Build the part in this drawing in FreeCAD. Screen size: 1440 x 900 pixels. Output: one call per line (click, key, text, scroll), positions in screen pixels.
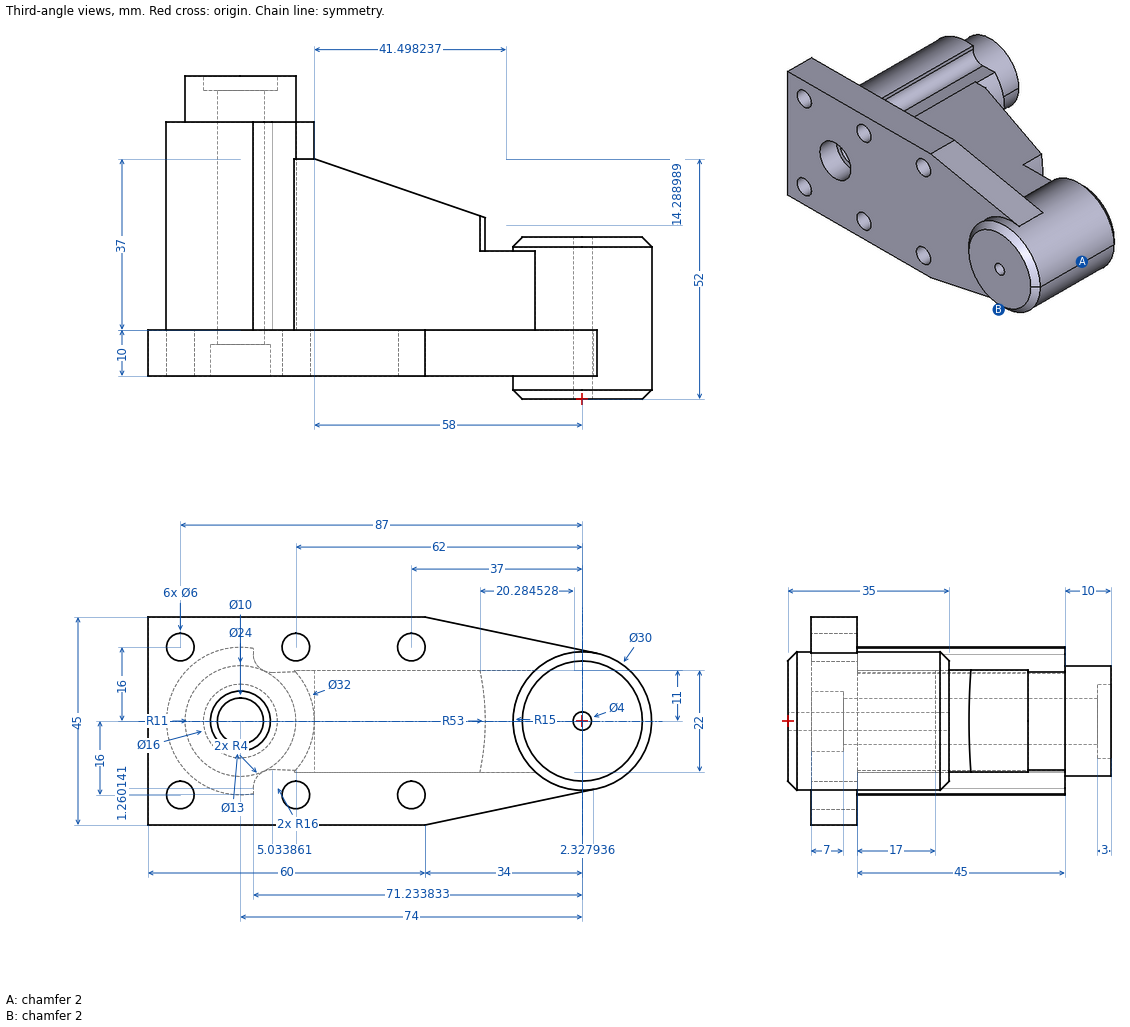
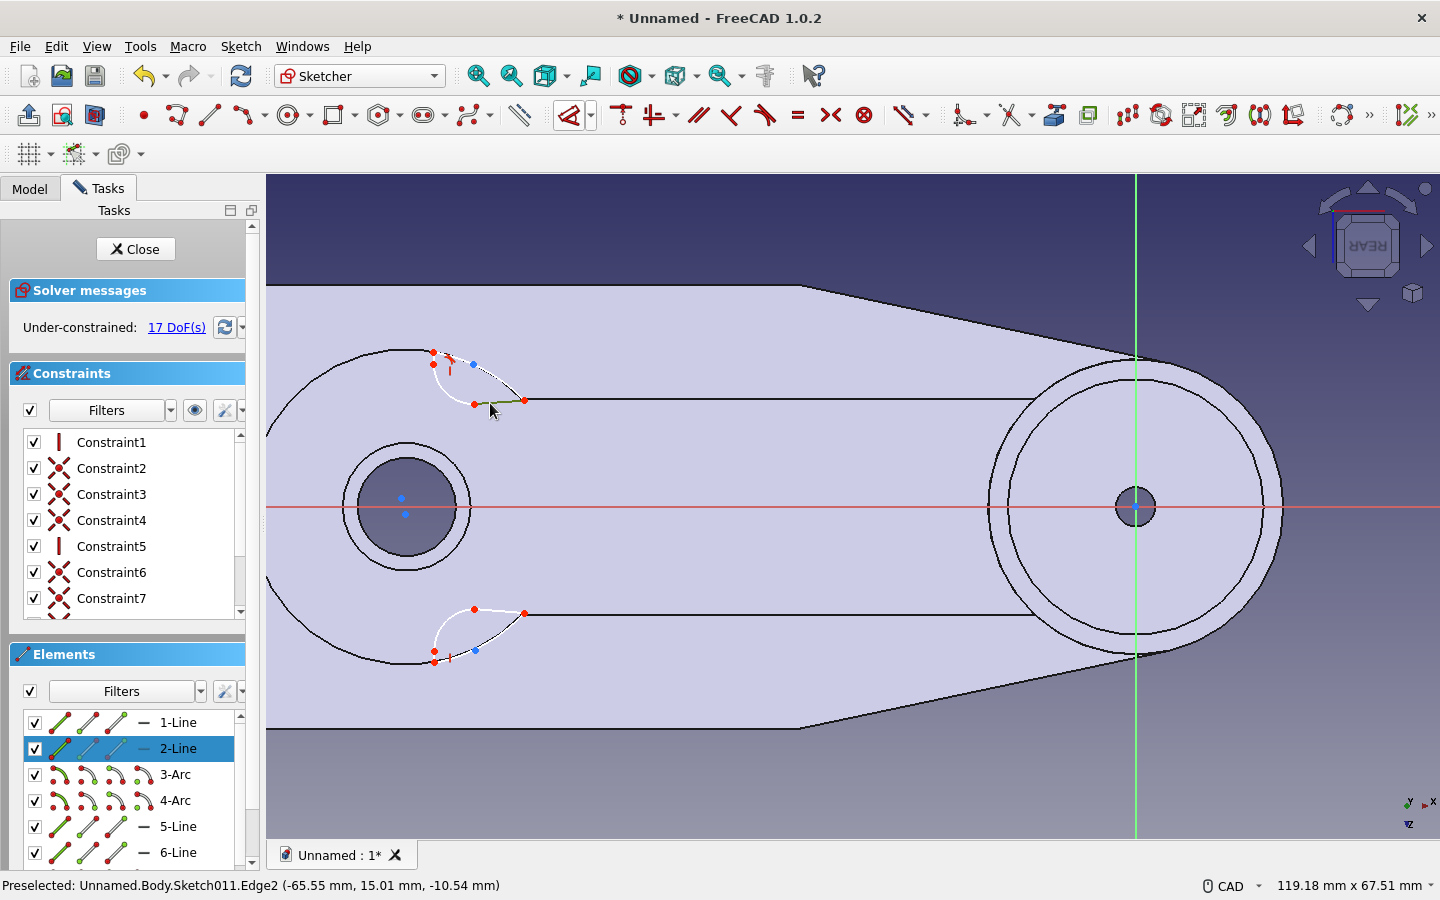
click(438, 383)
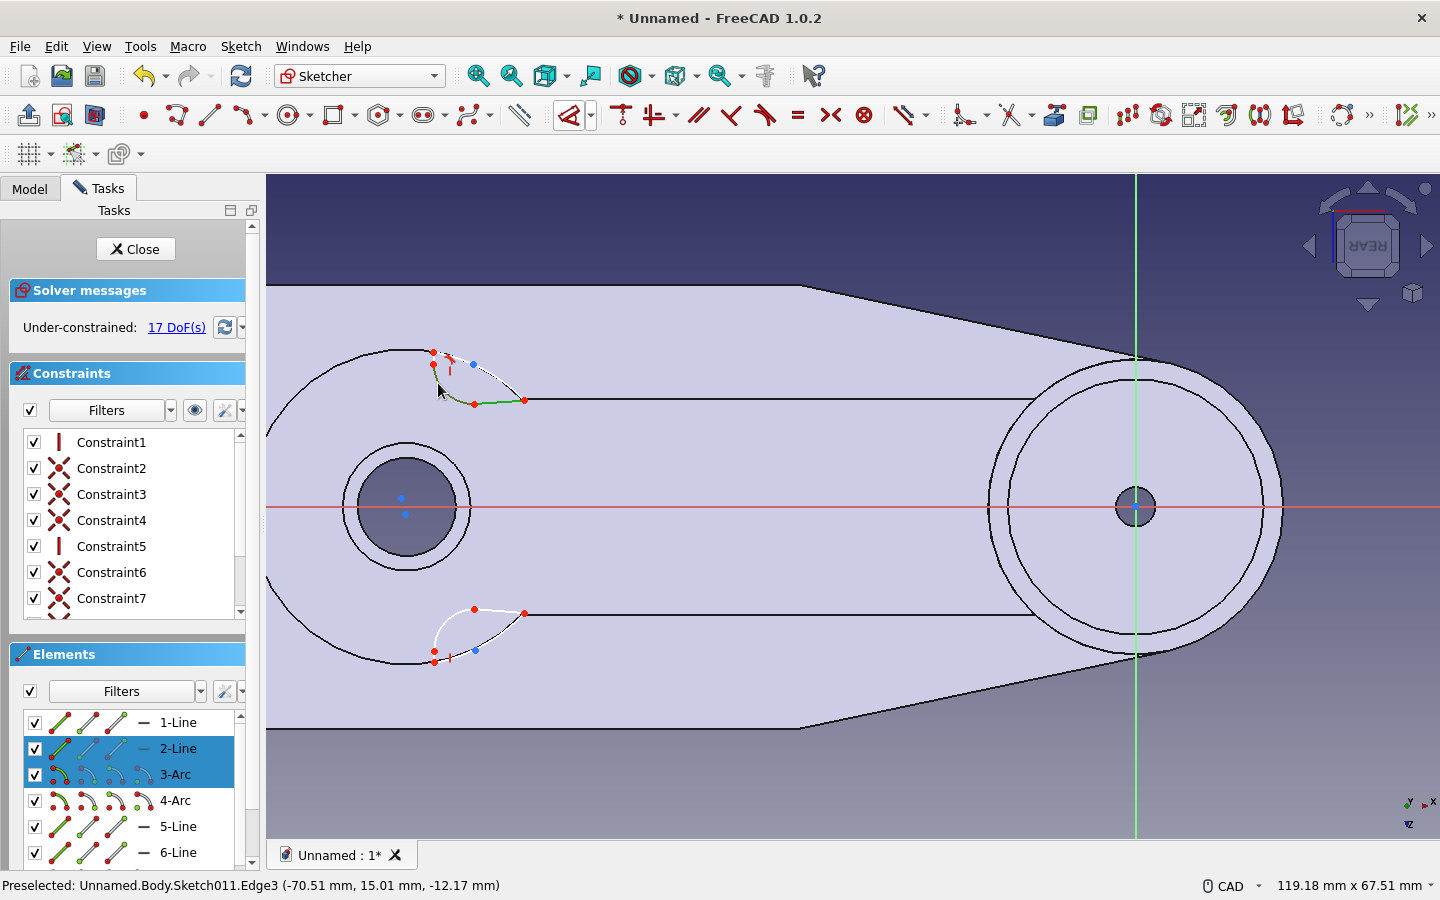
click(765, 116)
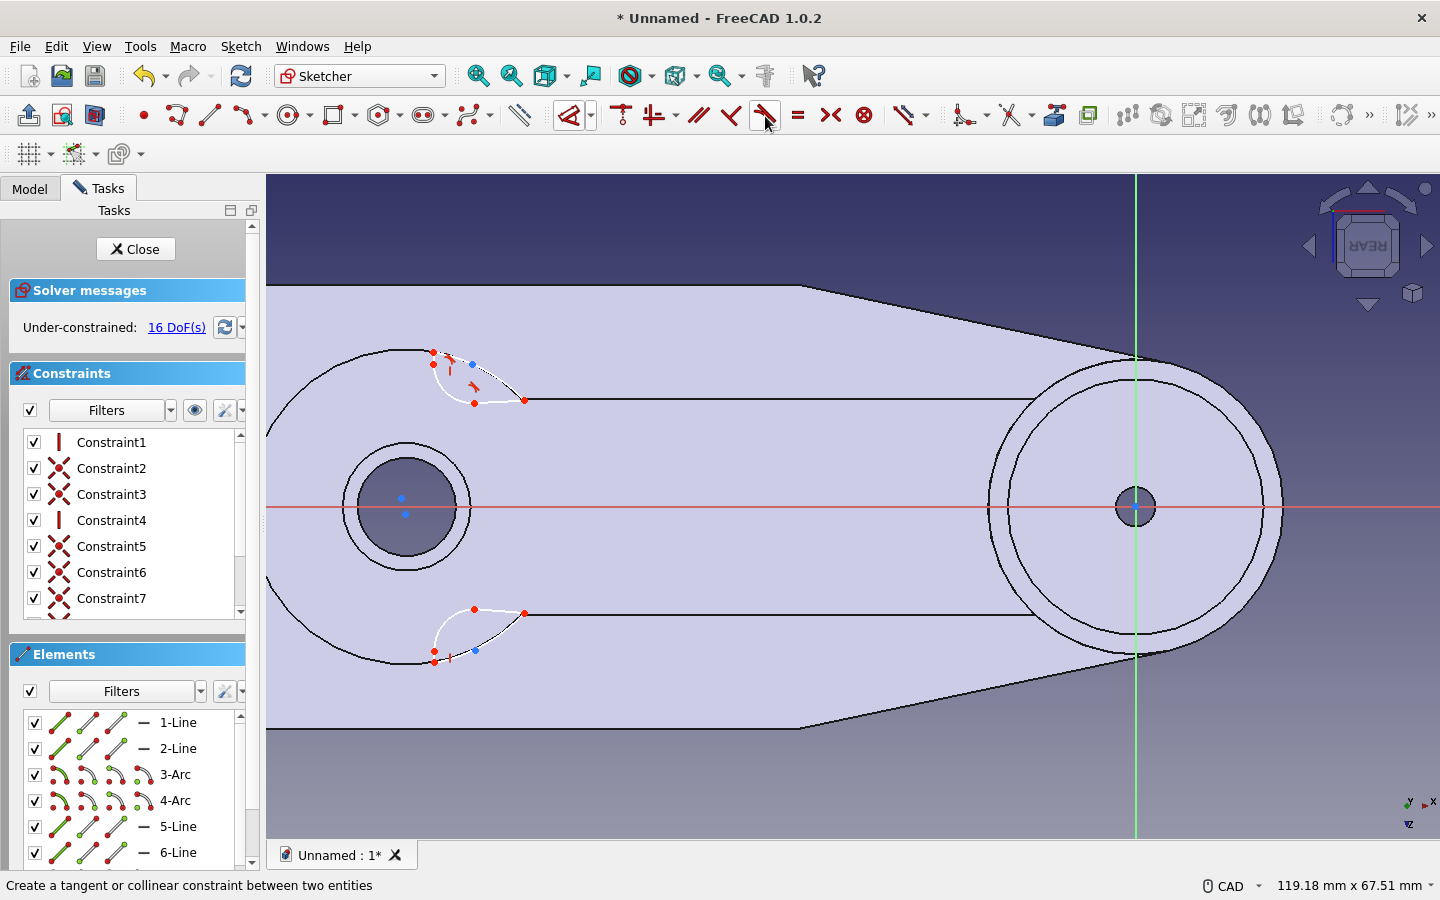
click(509, 612)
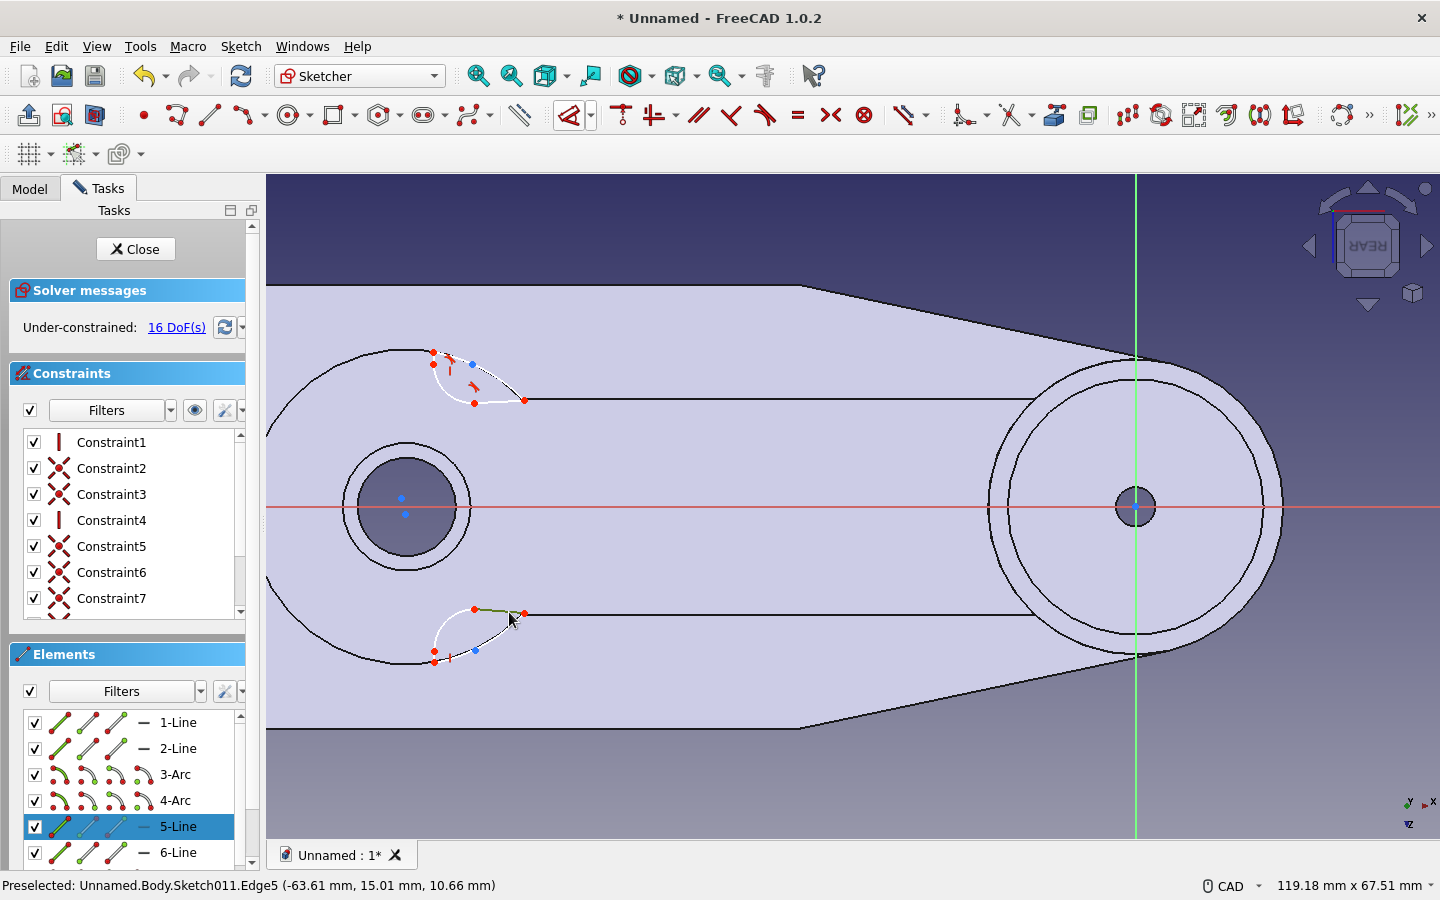
click(456, 614)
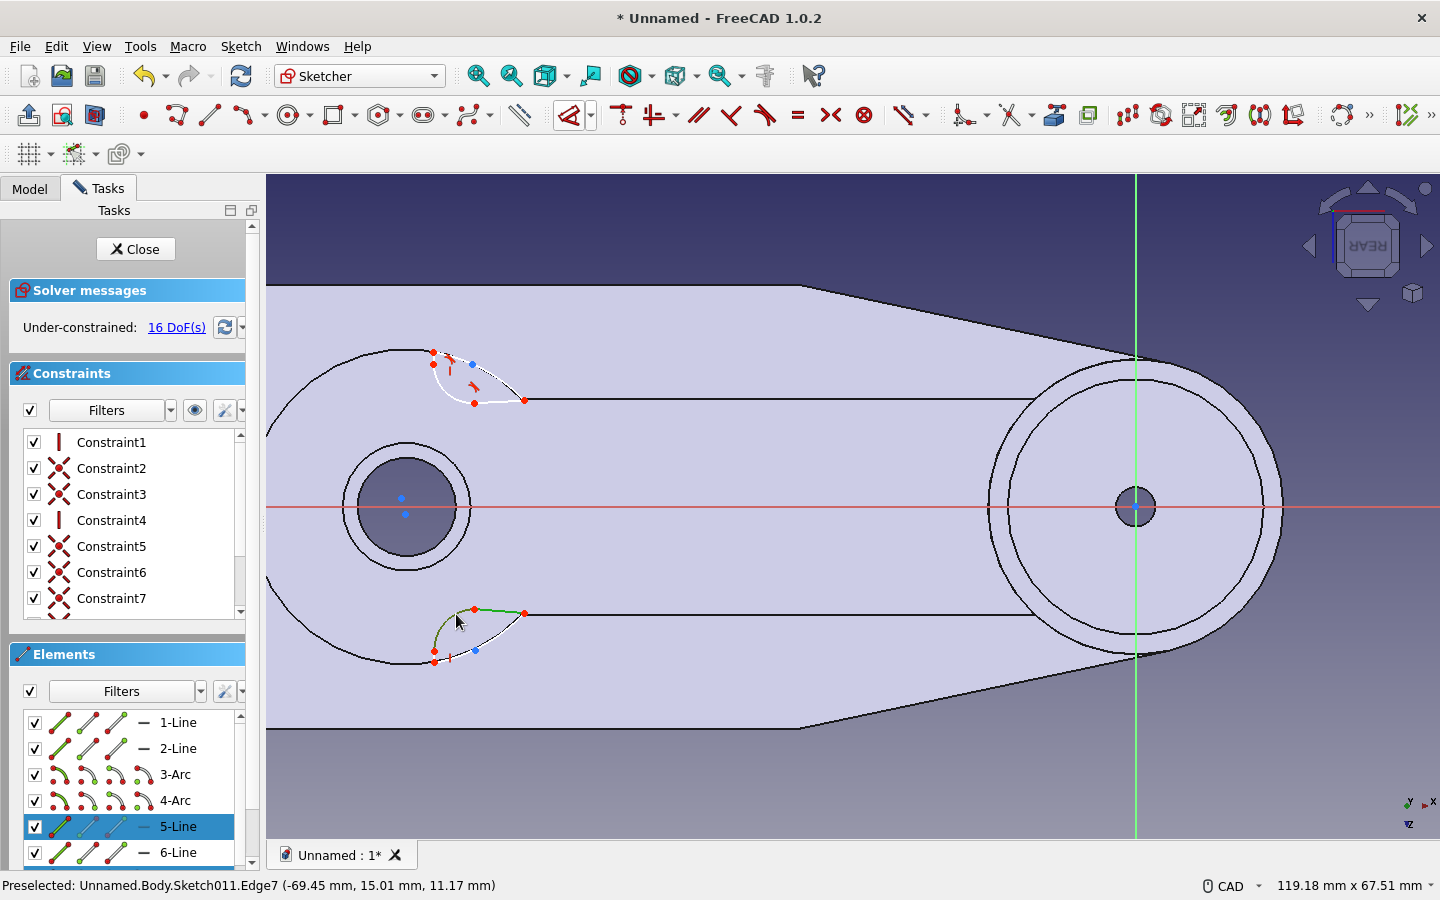
click(765, 116)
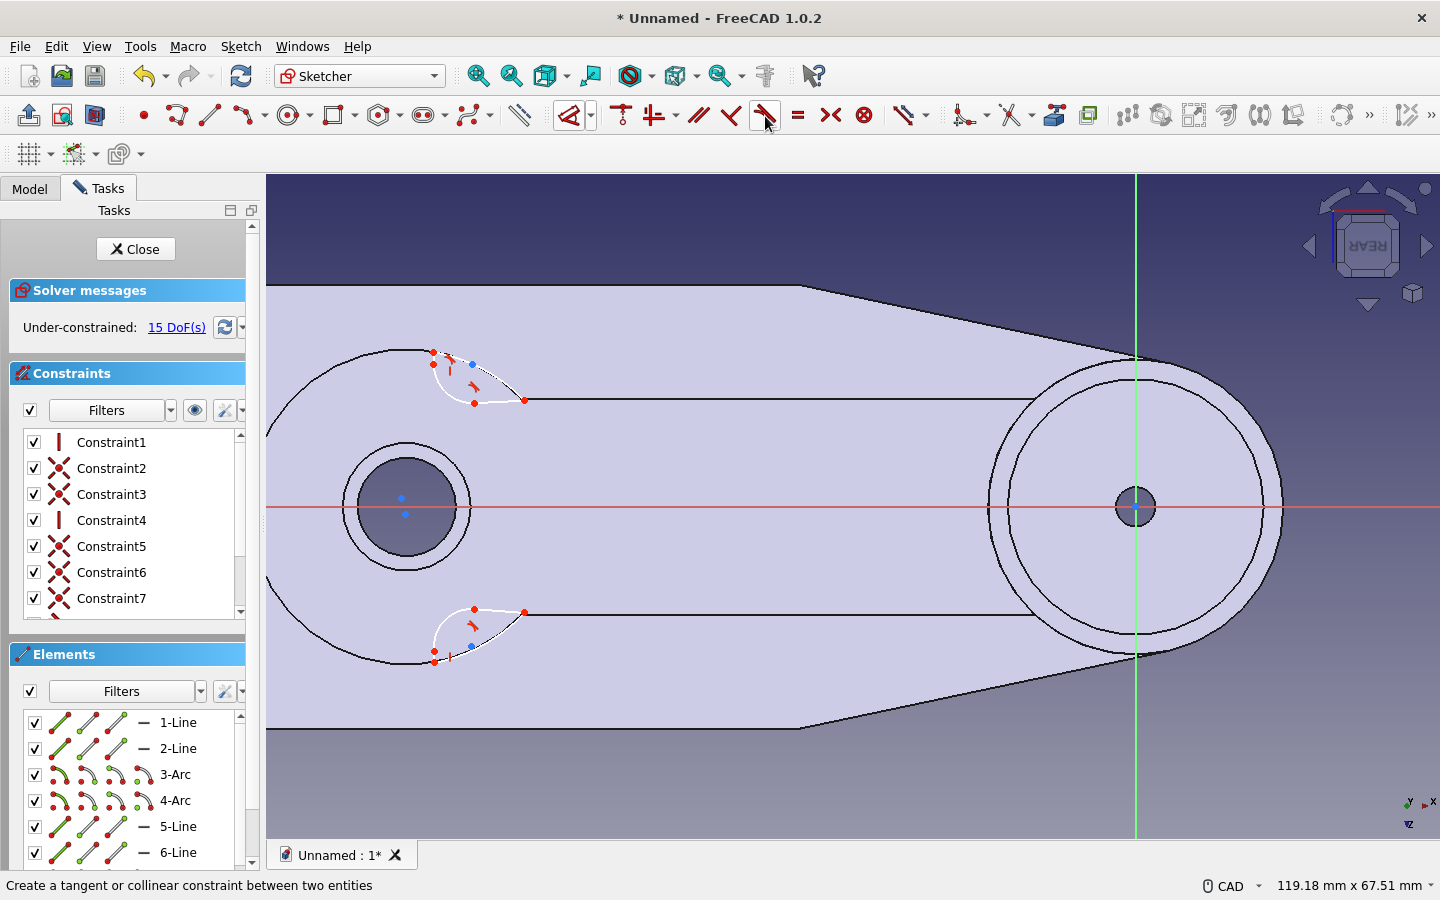
scroll(434, 657, up, 5)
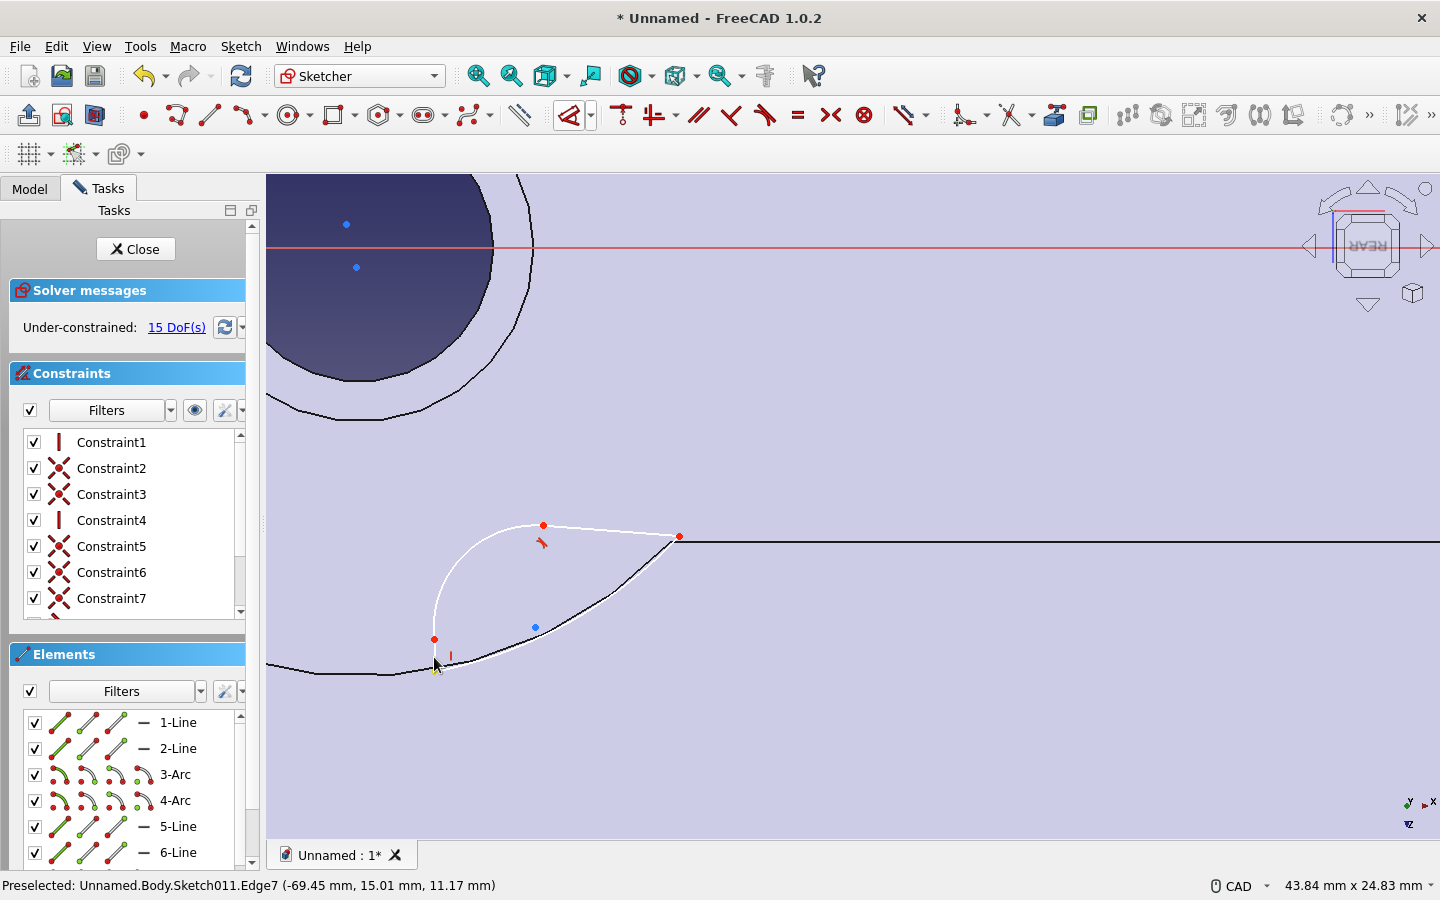
click(435, 656)